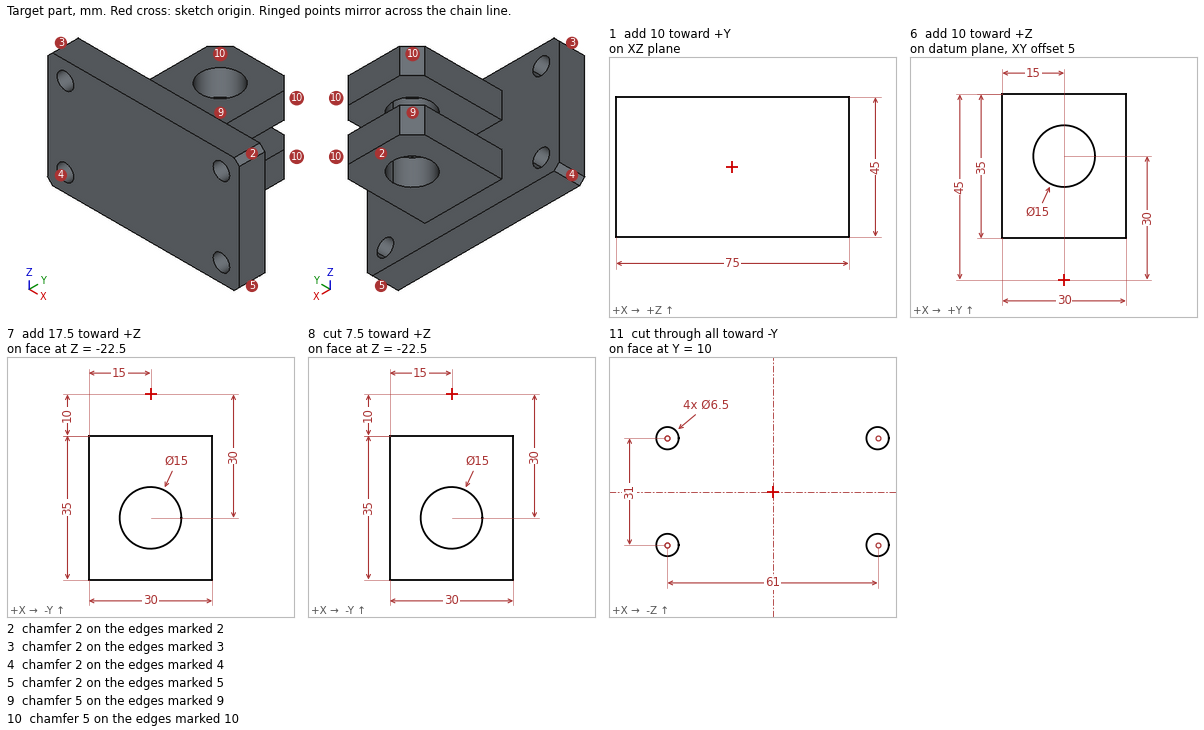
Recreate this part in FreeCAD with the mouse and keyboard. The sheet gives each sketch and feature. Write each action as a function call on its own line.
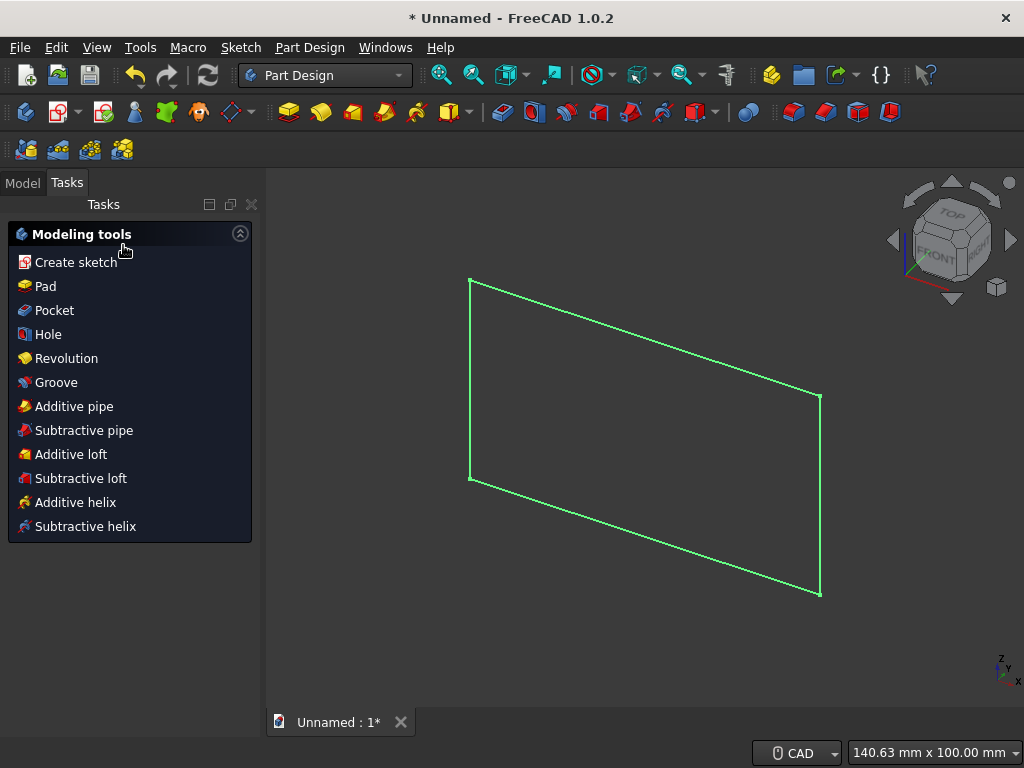
click(290, 112)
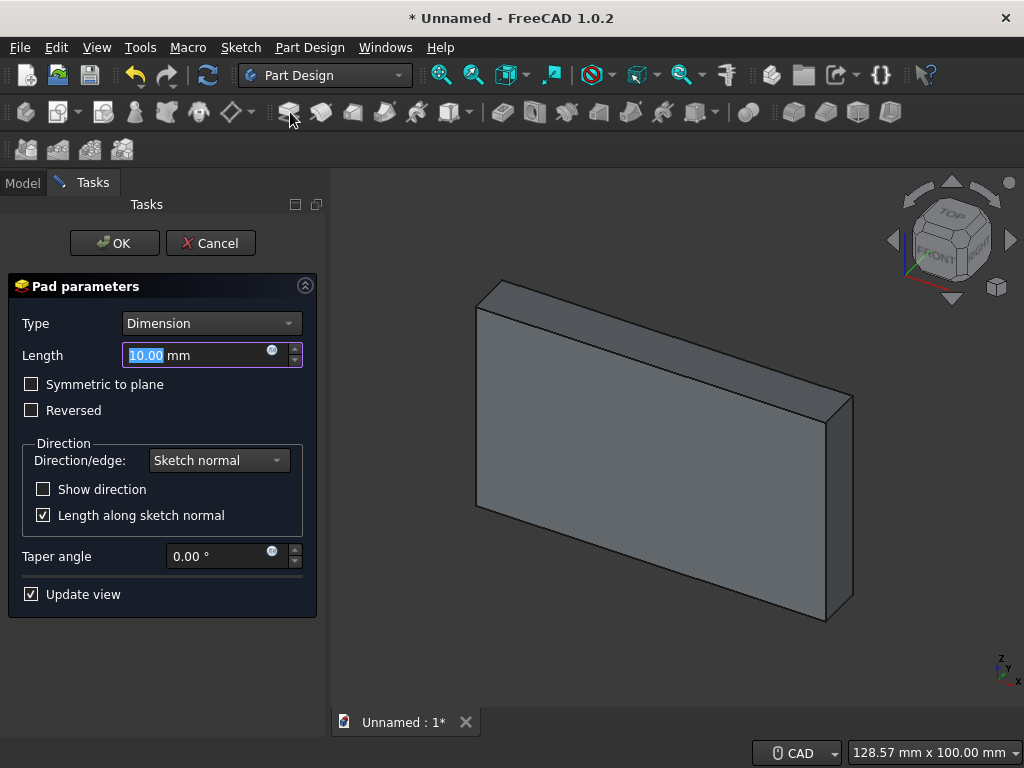
text(10)
key(Tab)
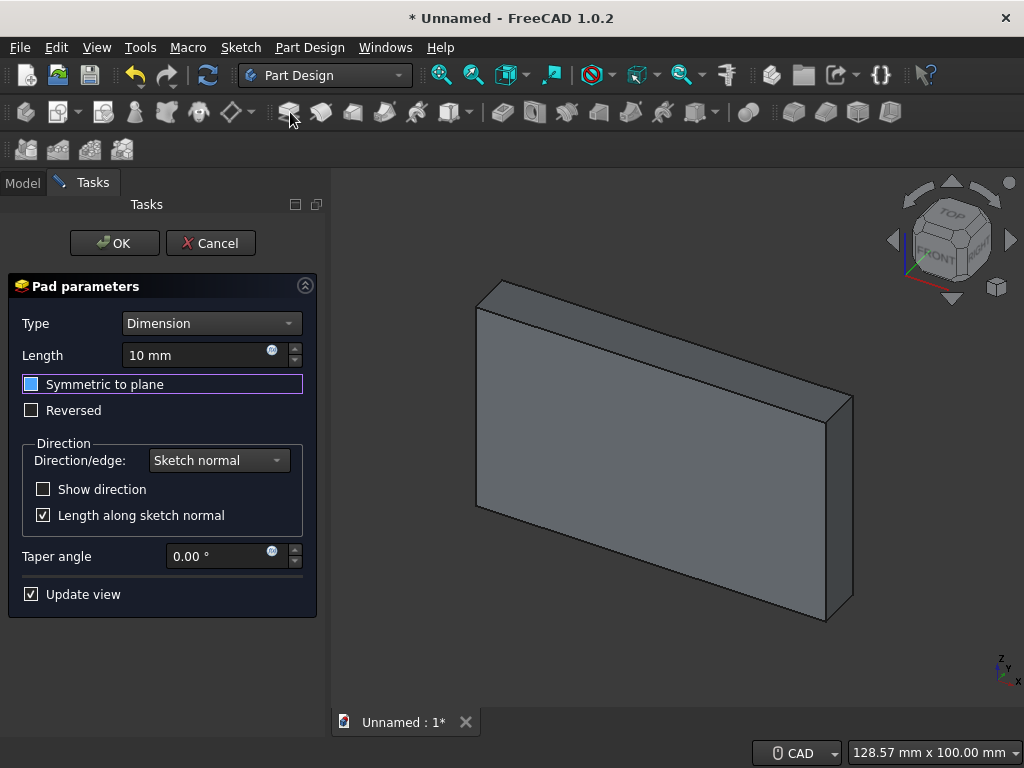
click(30, 410)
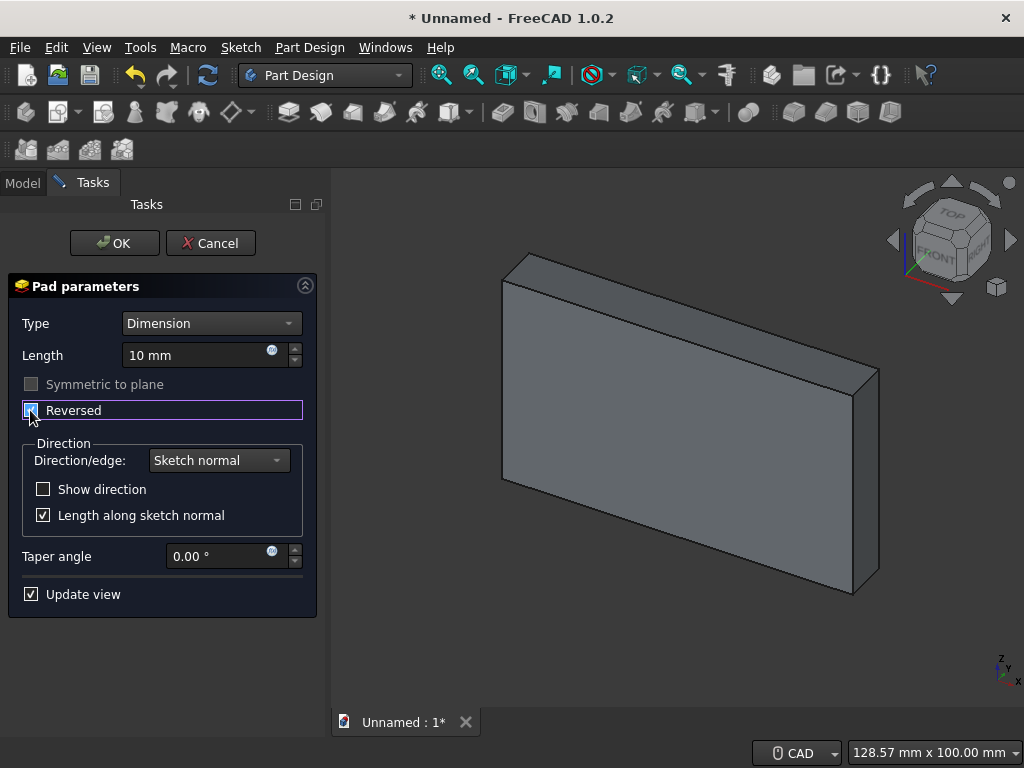
click(115, 243)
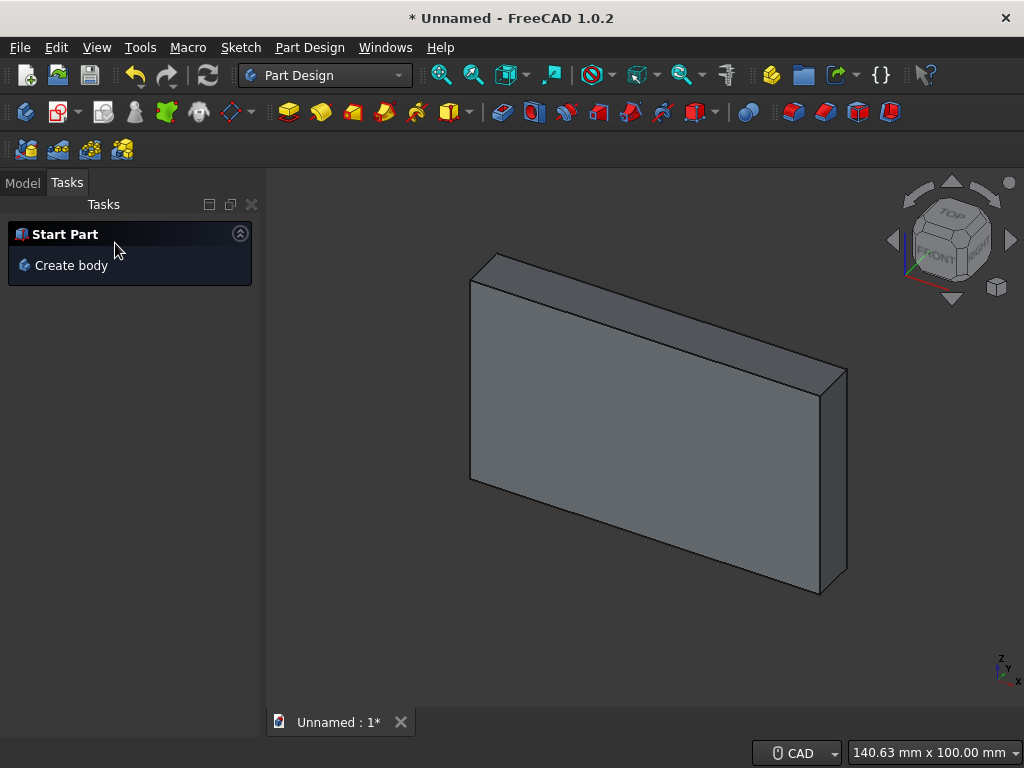
click(834, 382)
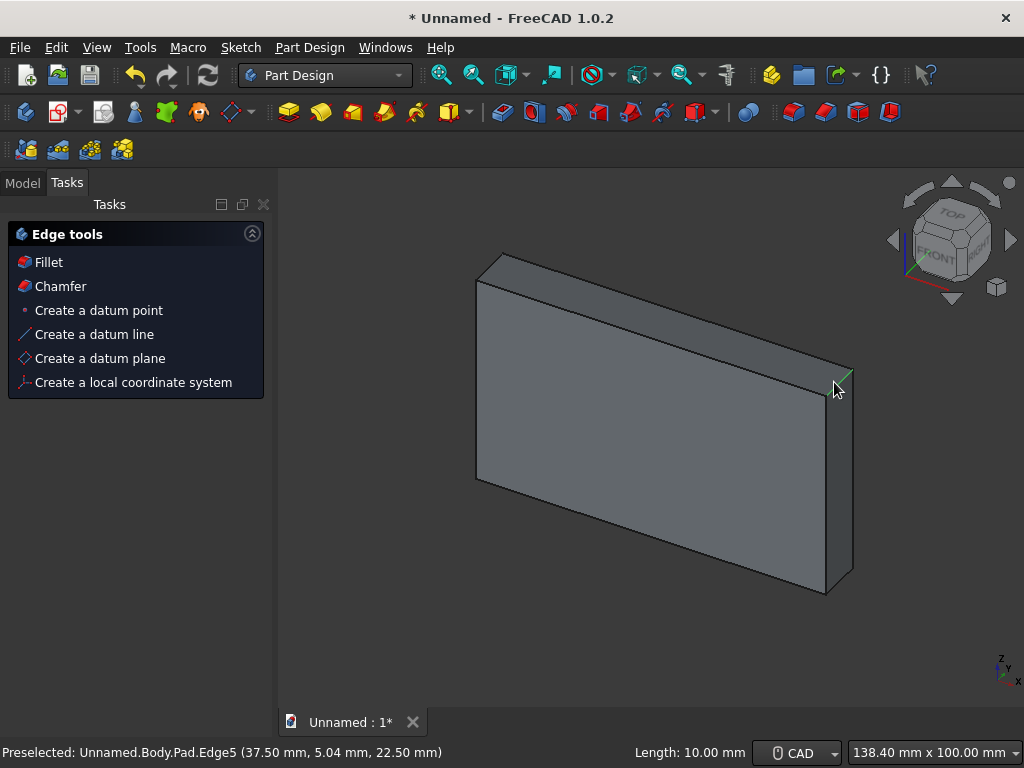
click(826, 112)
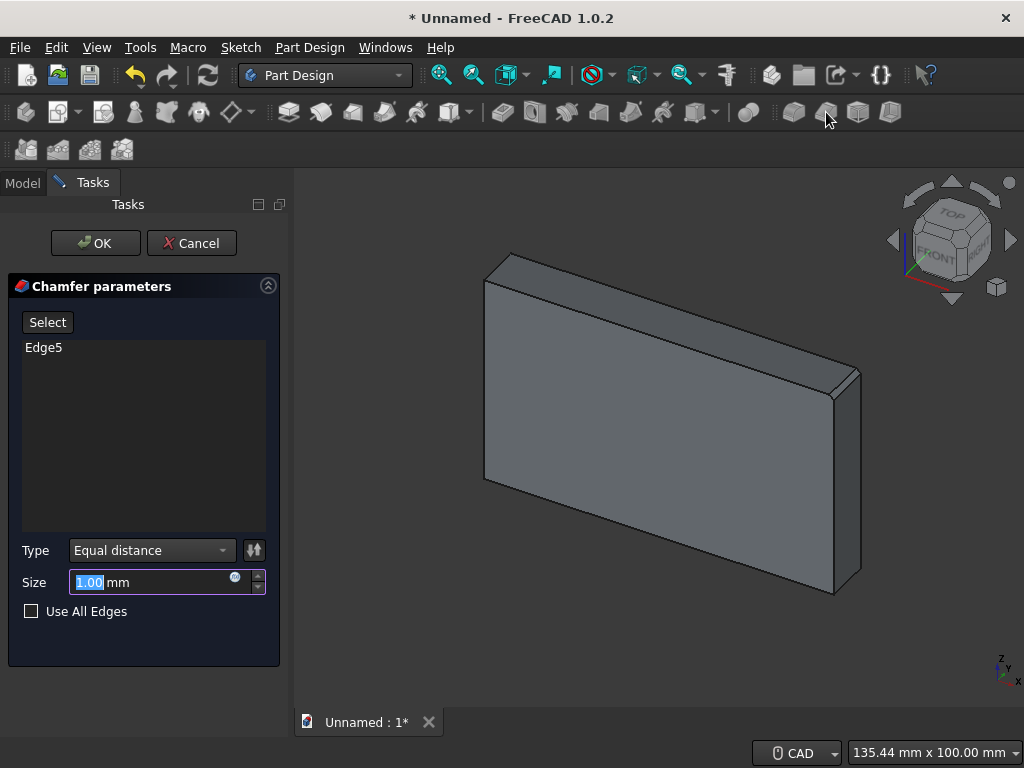
text(2)
key(Tab)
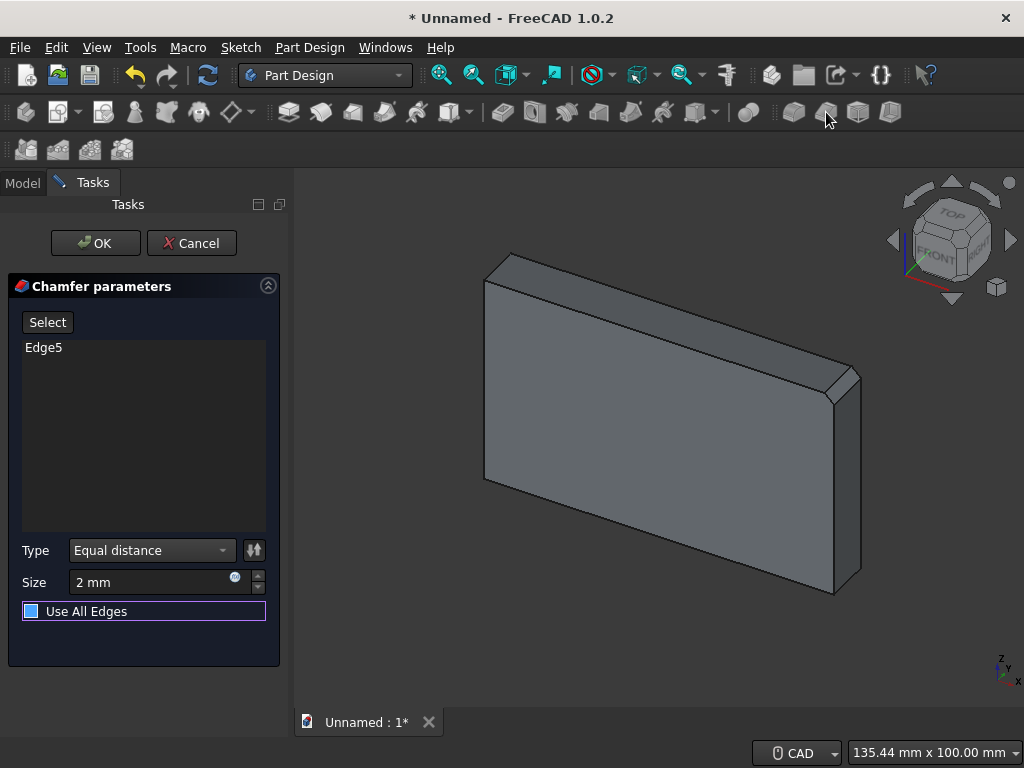
click(96, 243)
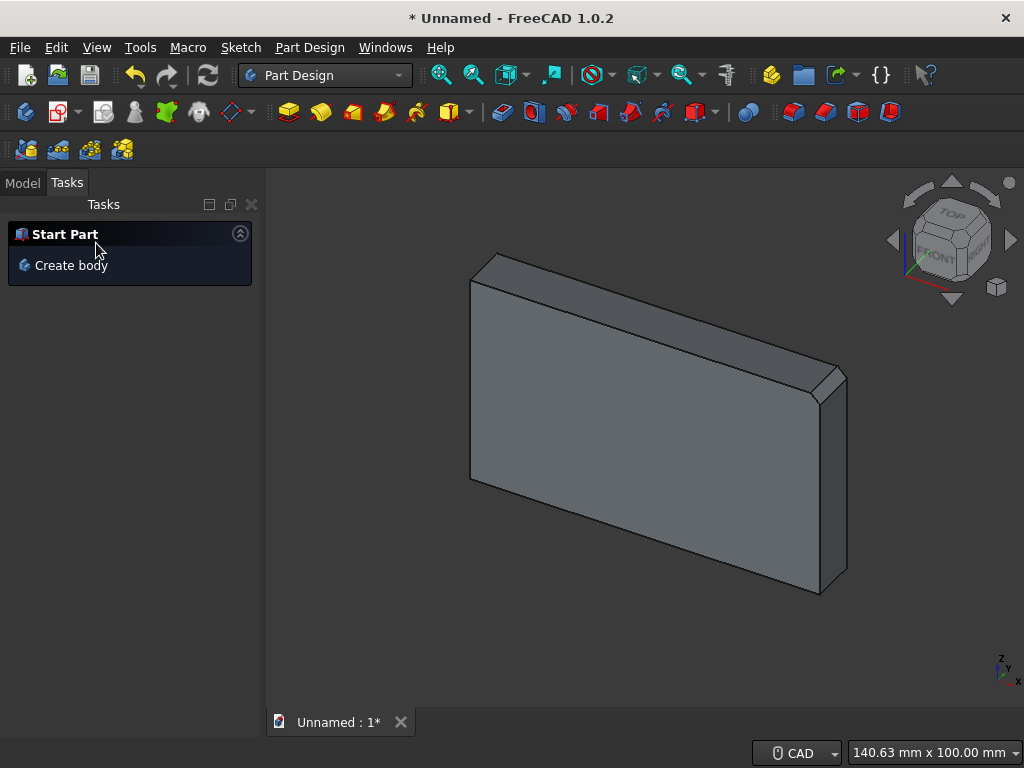
key(0)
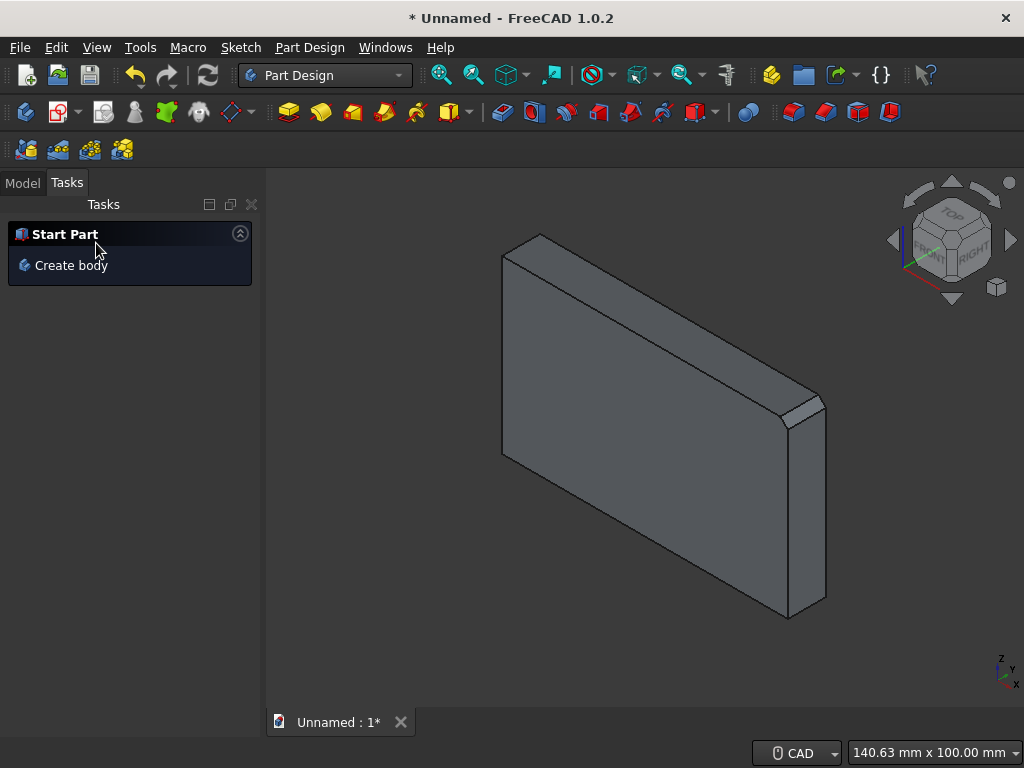
key(2)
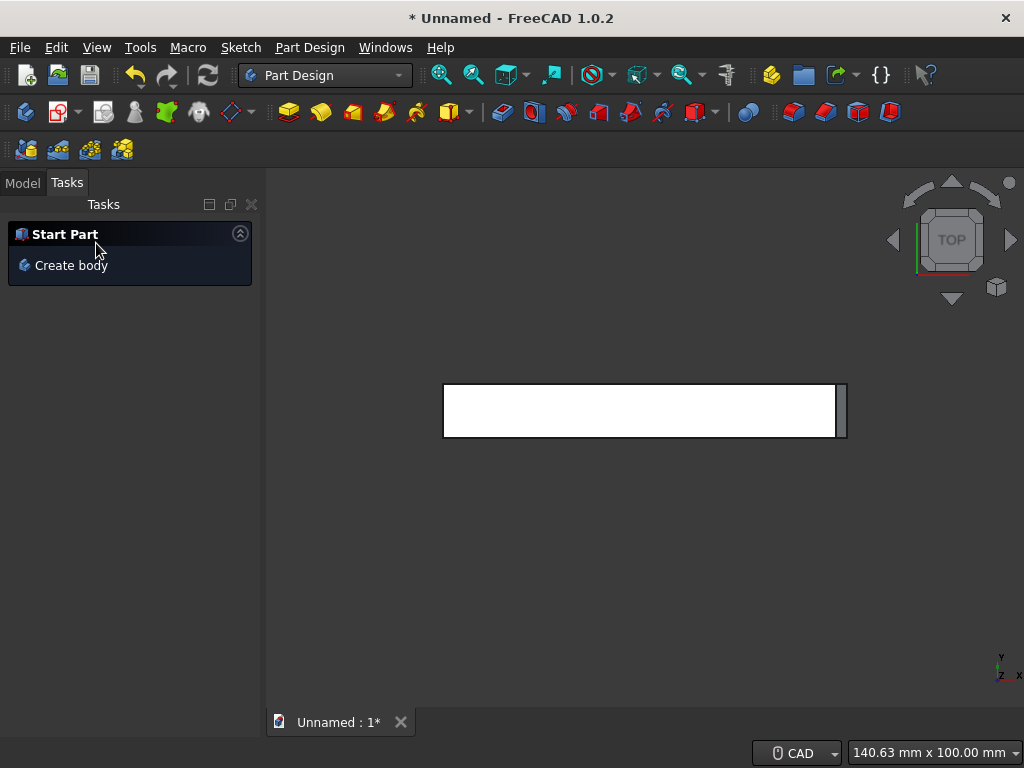
click(443, 410)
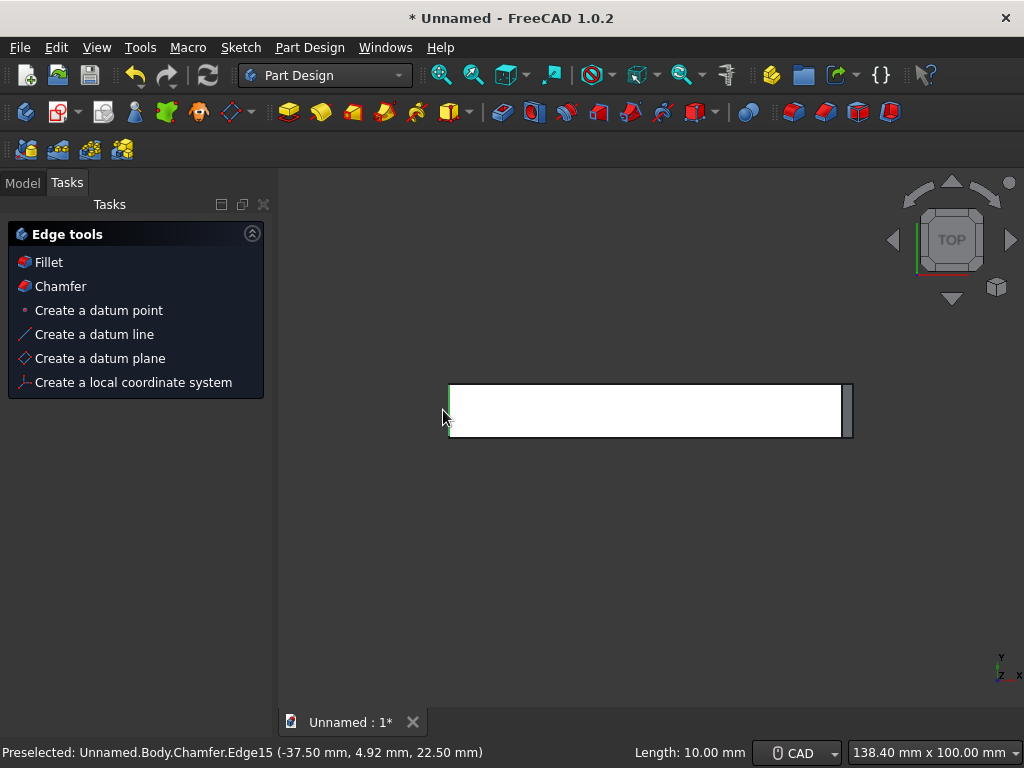
click(826, 112)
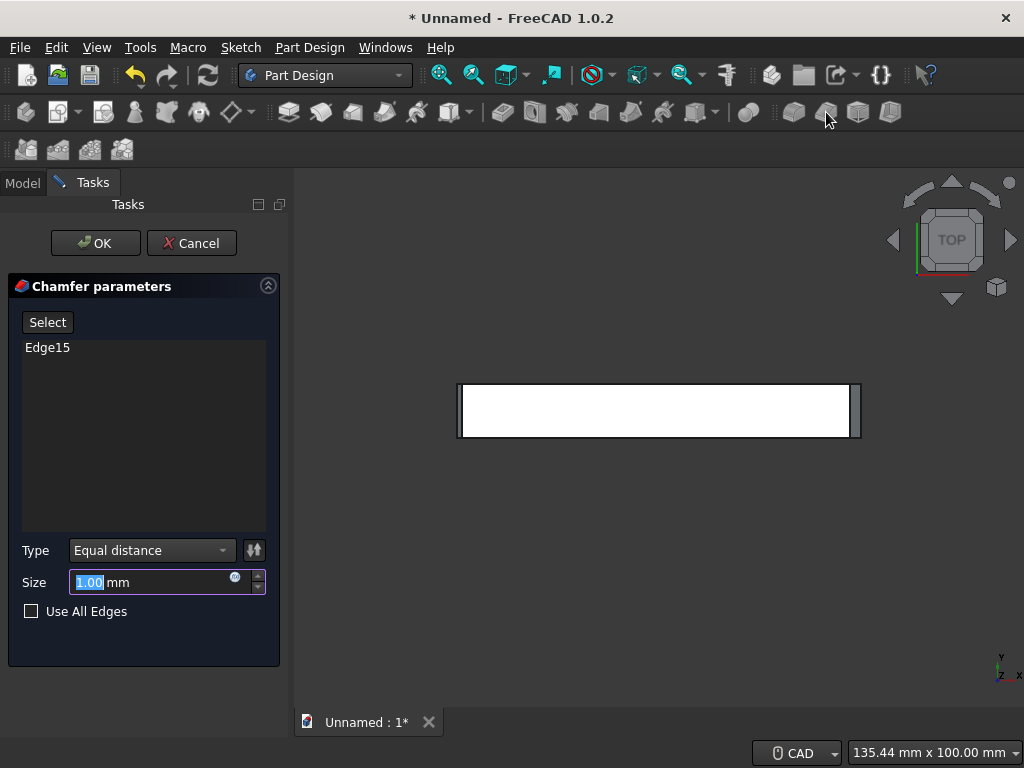
text(2)
key(Tab)